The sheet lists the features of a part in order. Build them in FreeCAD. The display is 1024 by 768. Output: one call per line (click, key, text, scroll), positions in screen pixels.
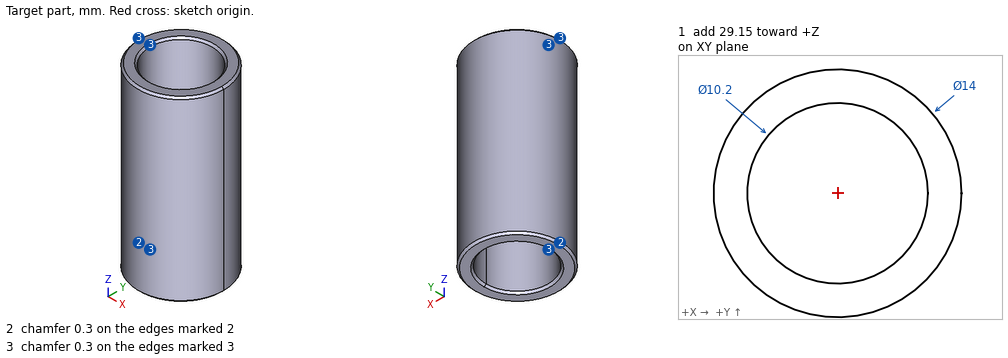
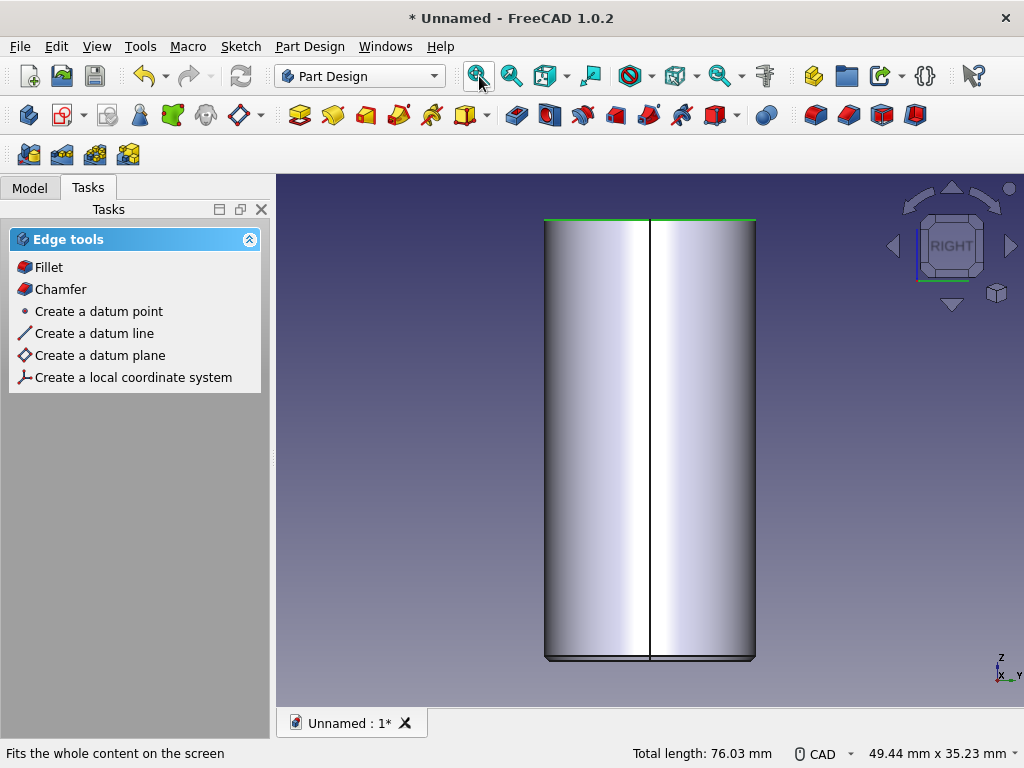
key(5)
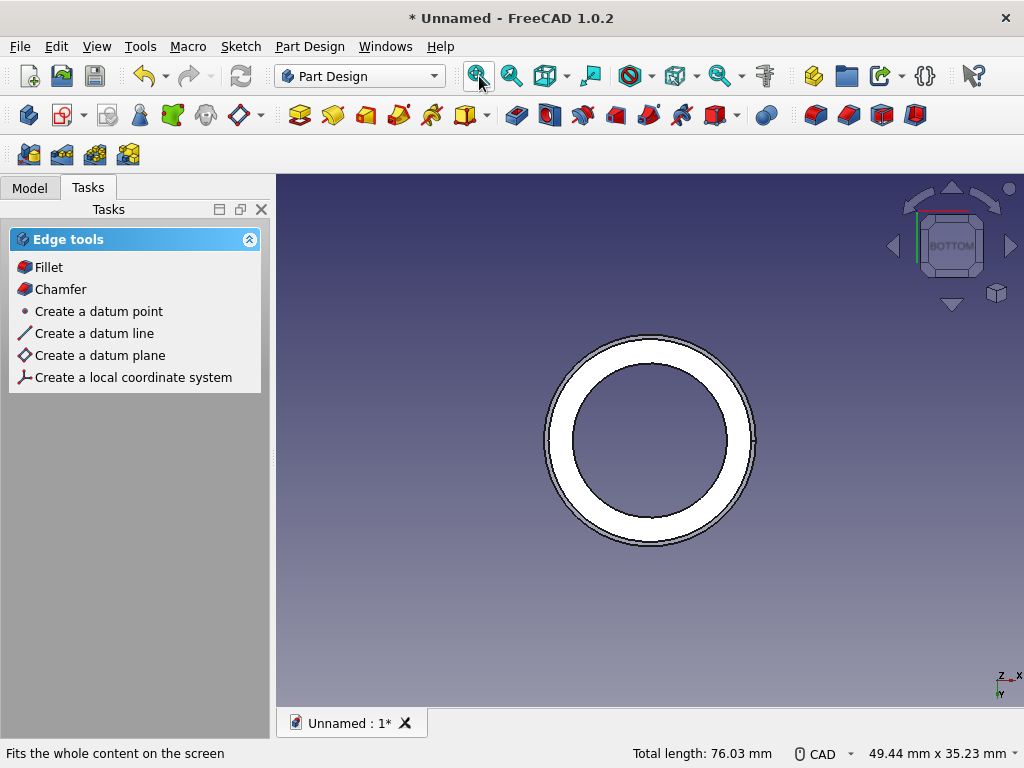
click(479, 76)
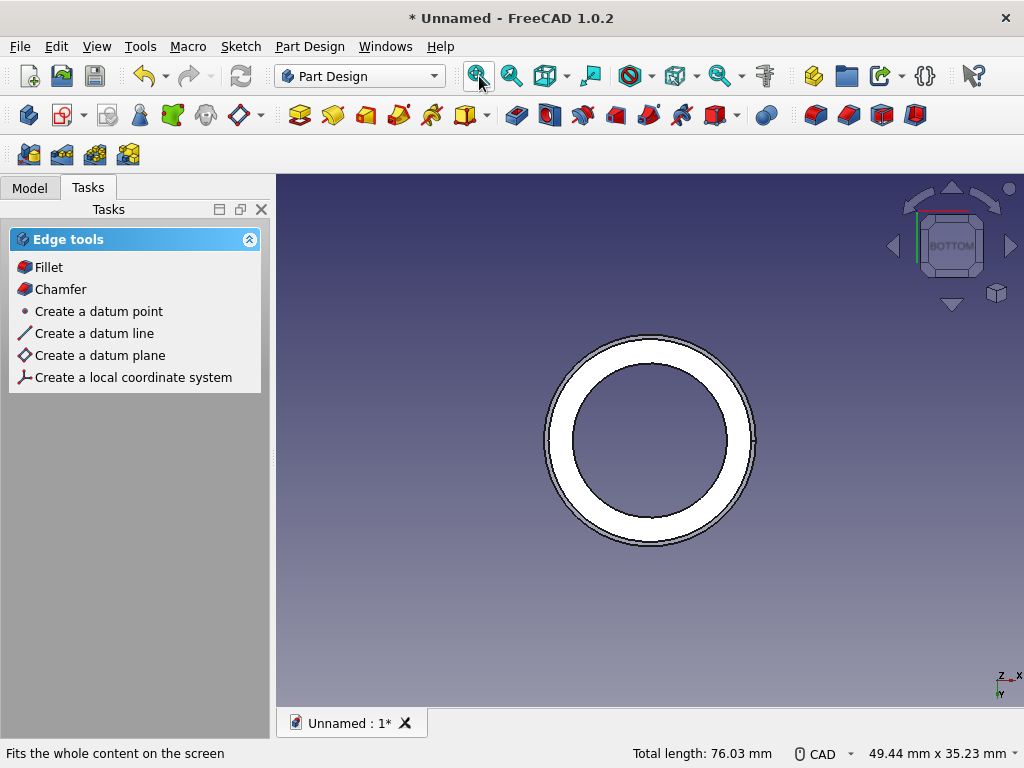
click(573, 439, ctrl)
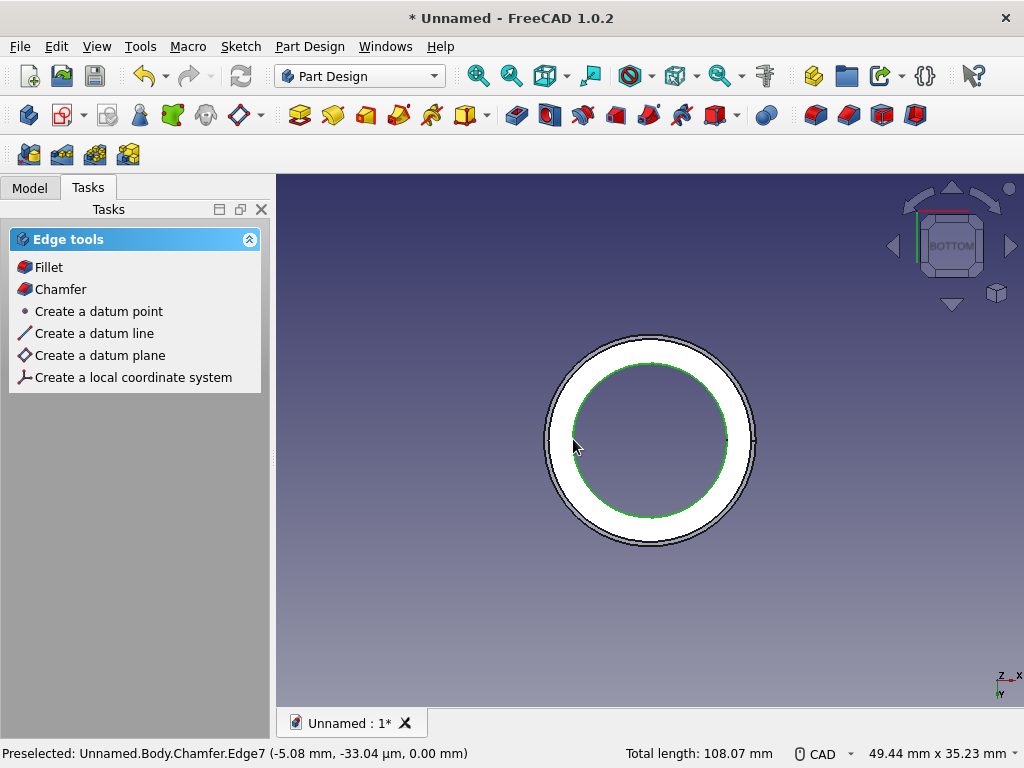
click(849, 116)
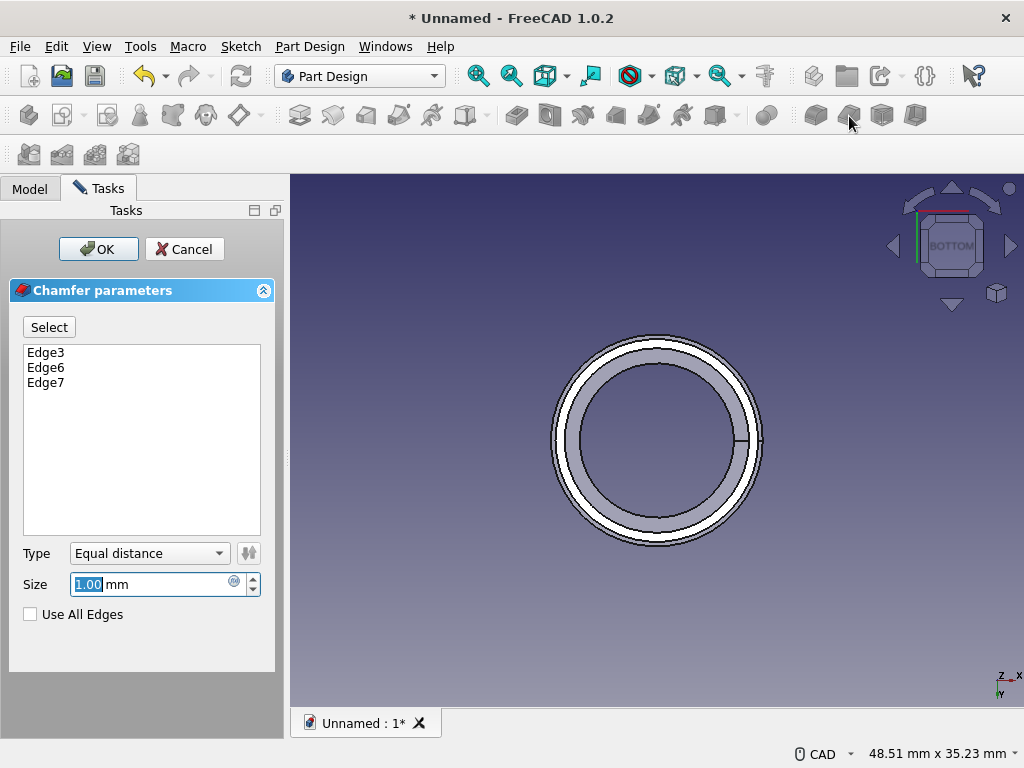
text(0.3)
key(Tab)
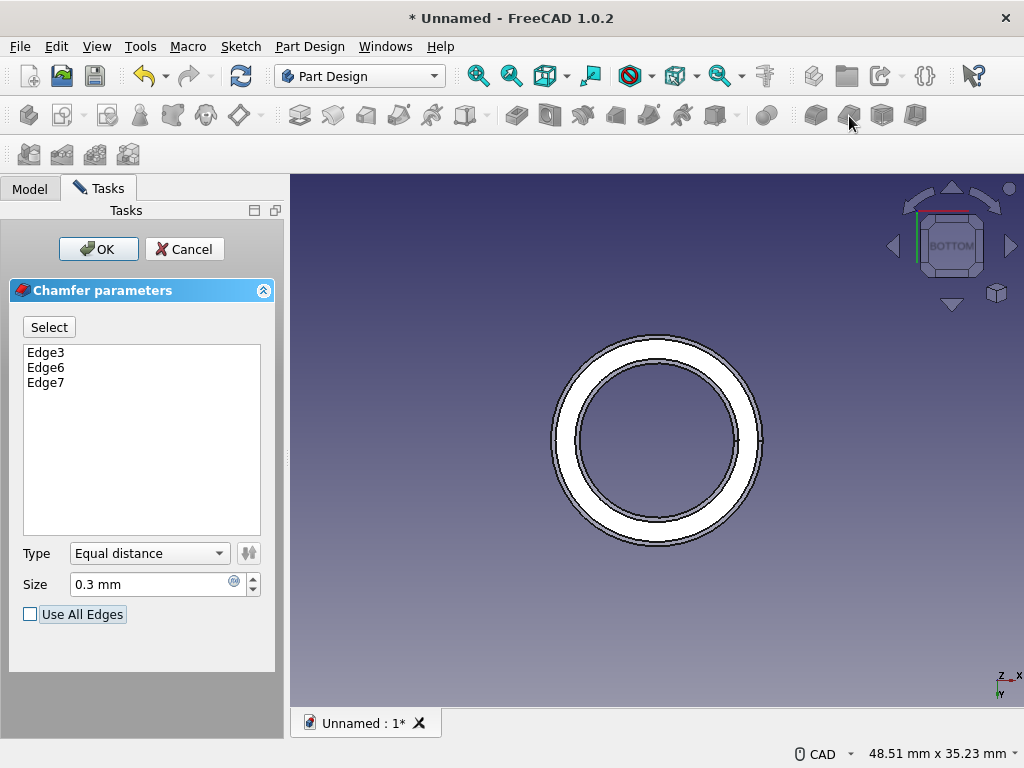
click(99, 249)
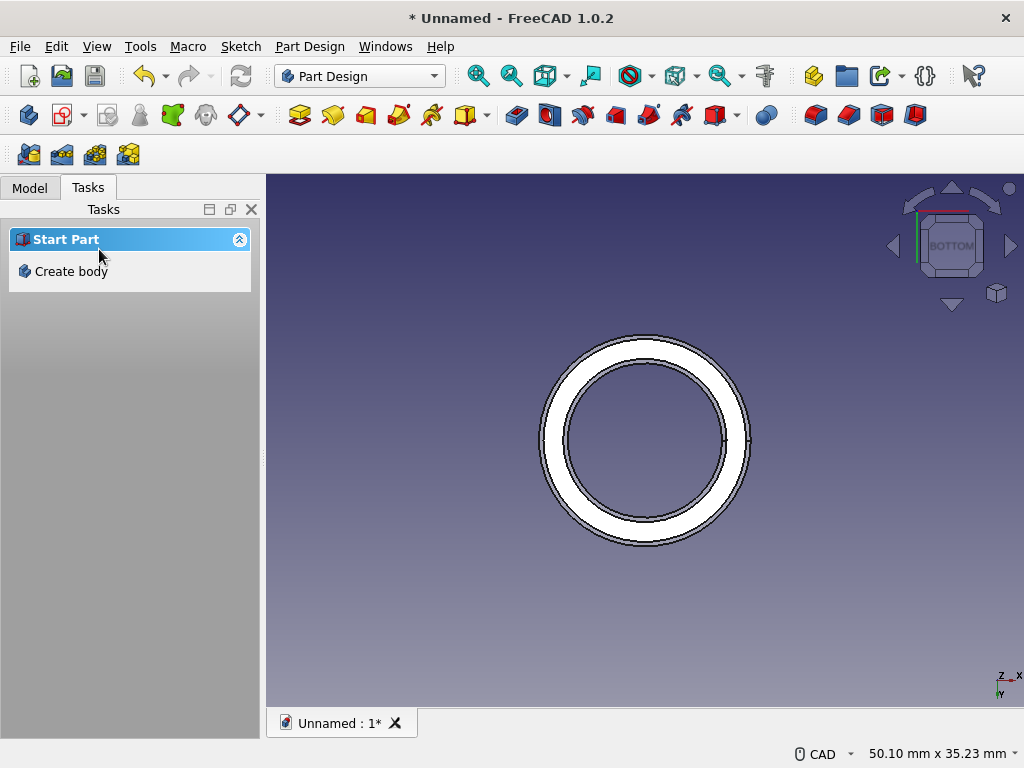
key(0)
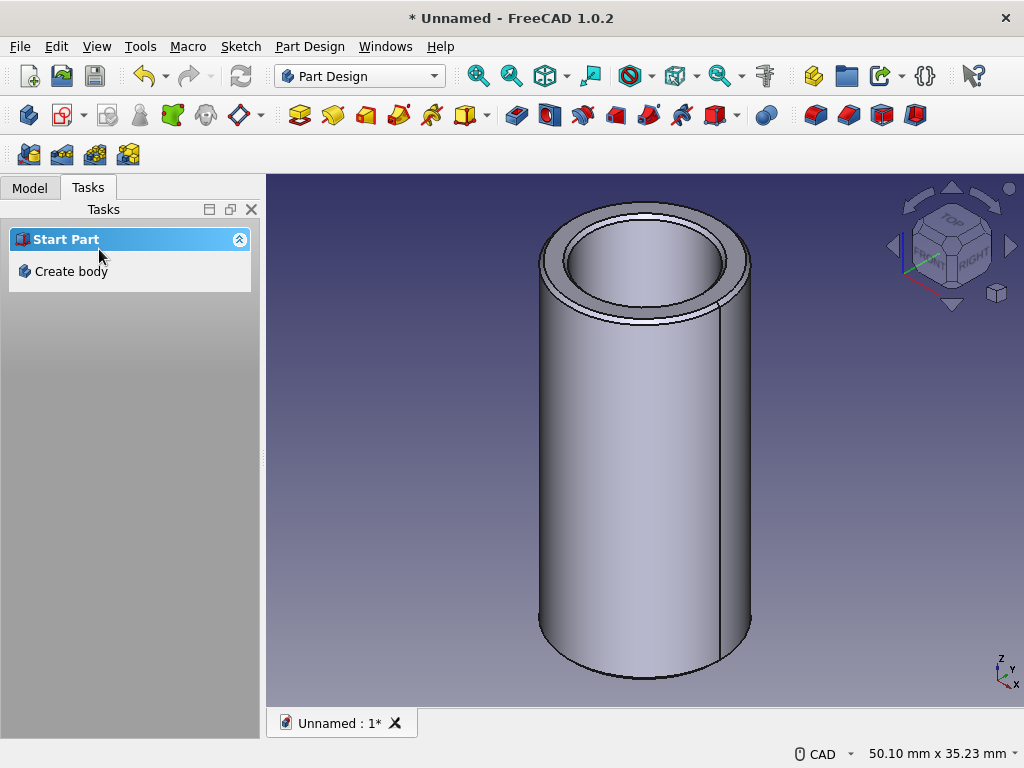
key(v)
key(f)